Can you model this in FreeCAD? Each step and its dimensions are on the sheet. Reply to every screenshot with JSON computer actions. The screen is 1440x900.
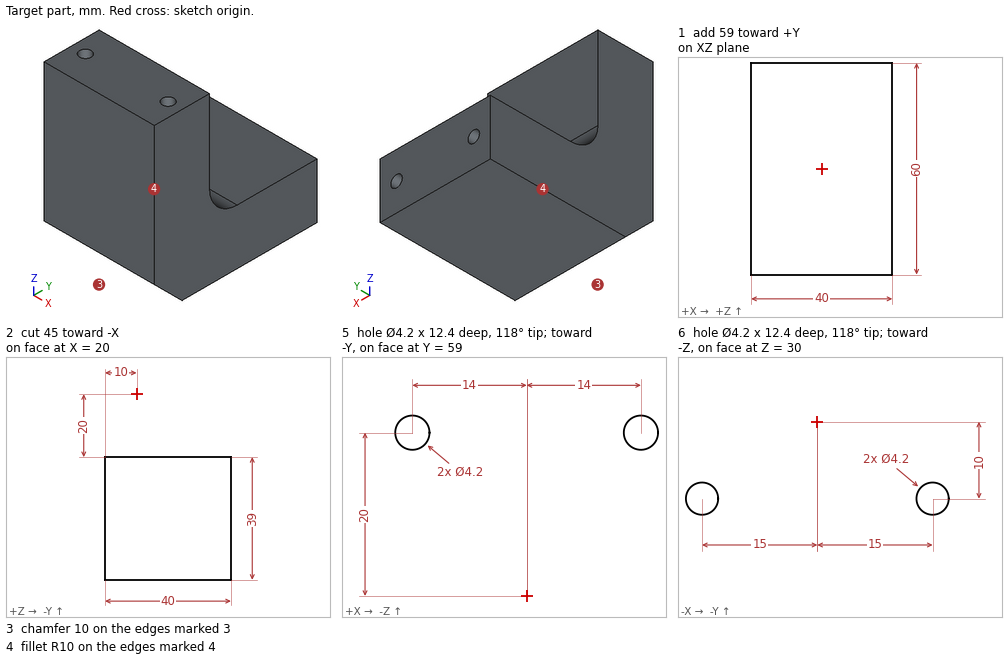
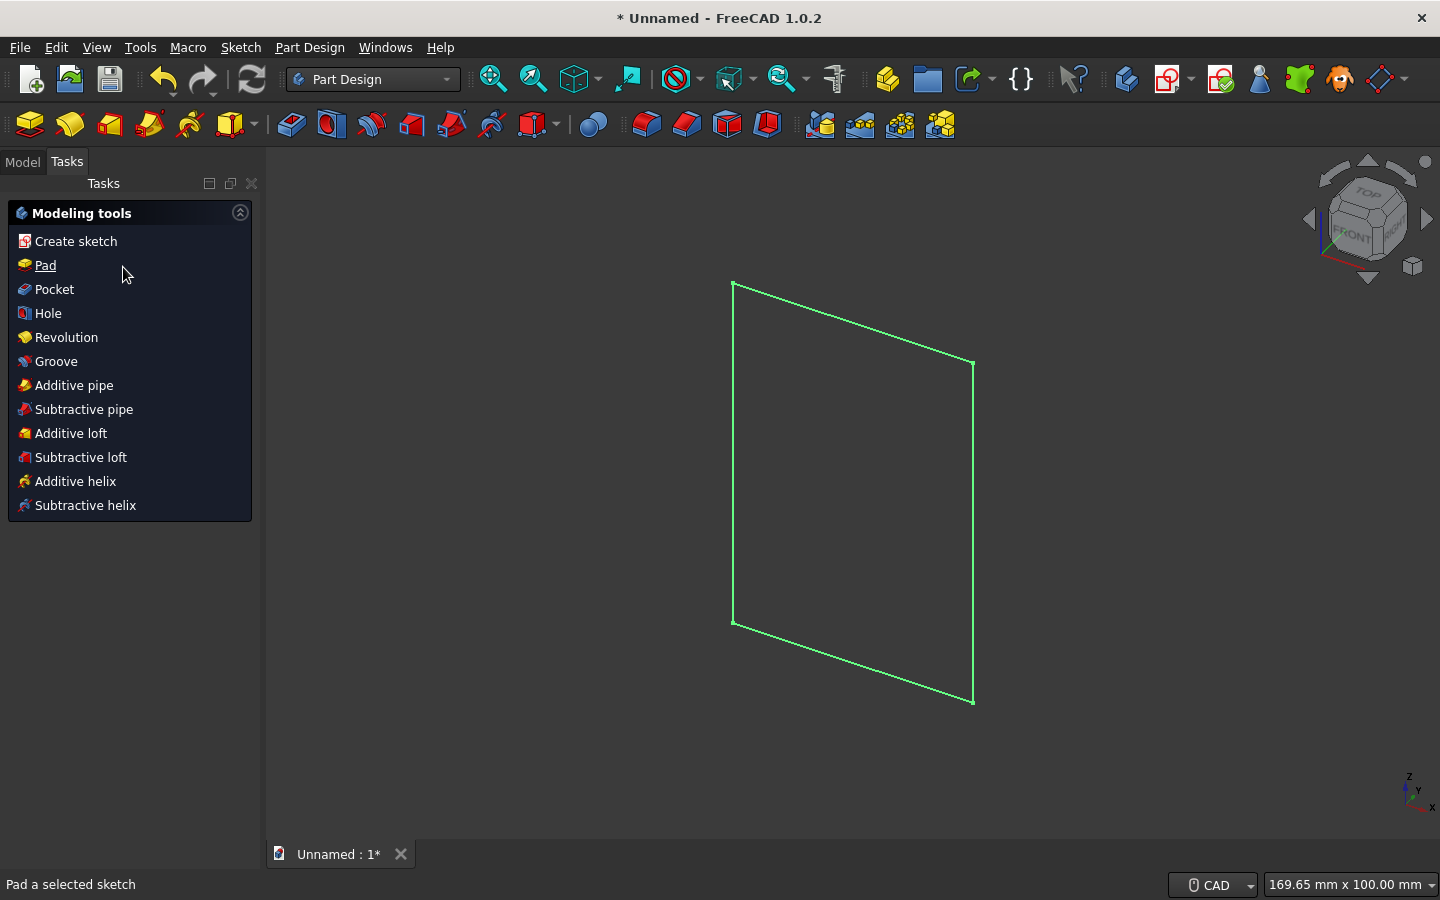
{"action": "left_click", "coordinate": [30, 124]}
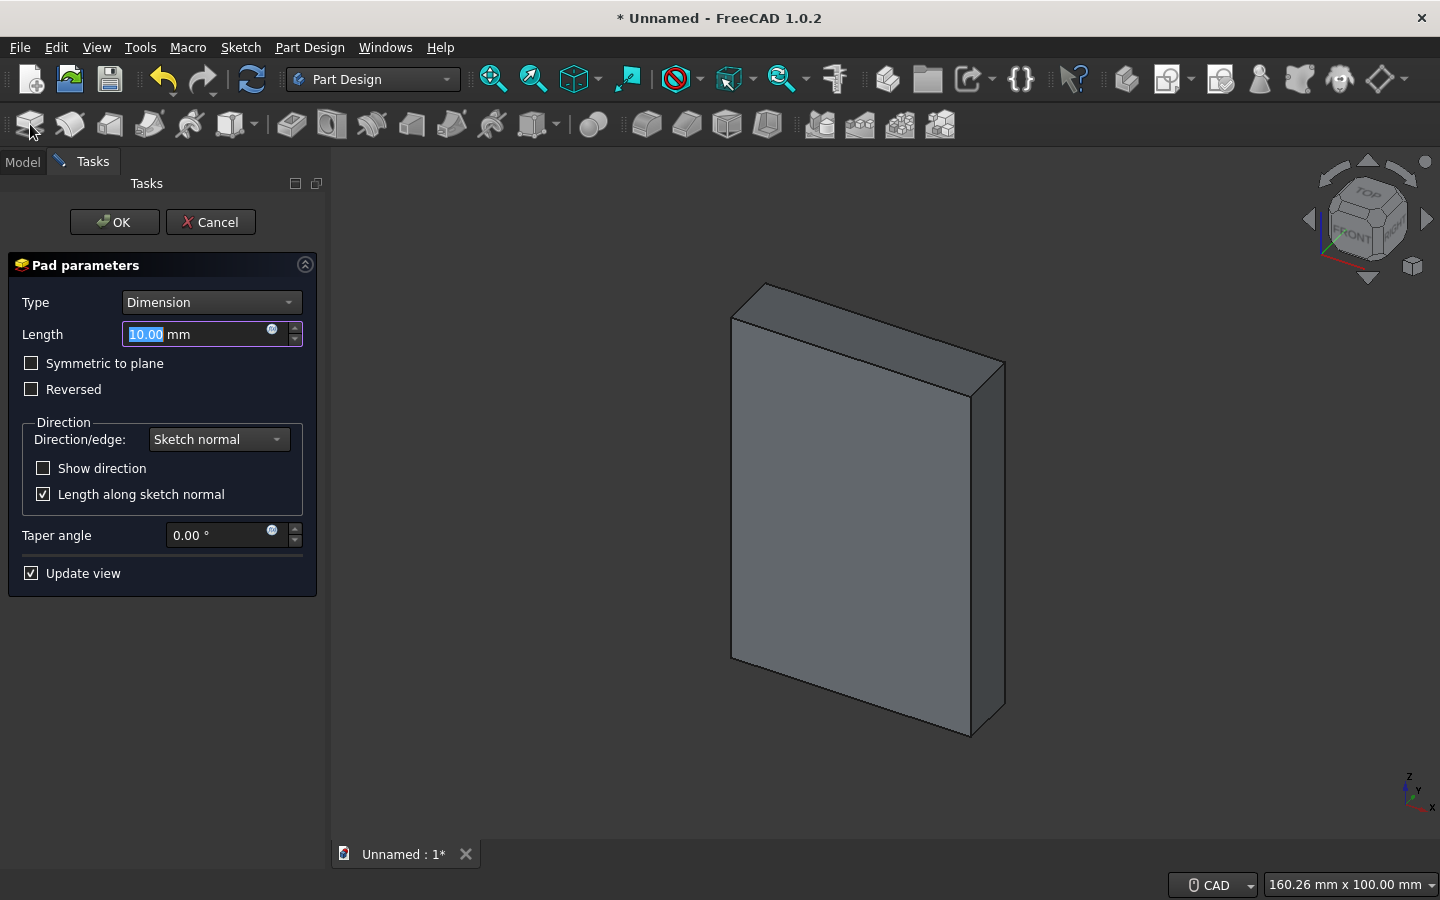
{"action": "type", "text": "59"}
{"action": "key", "text": "Tab"}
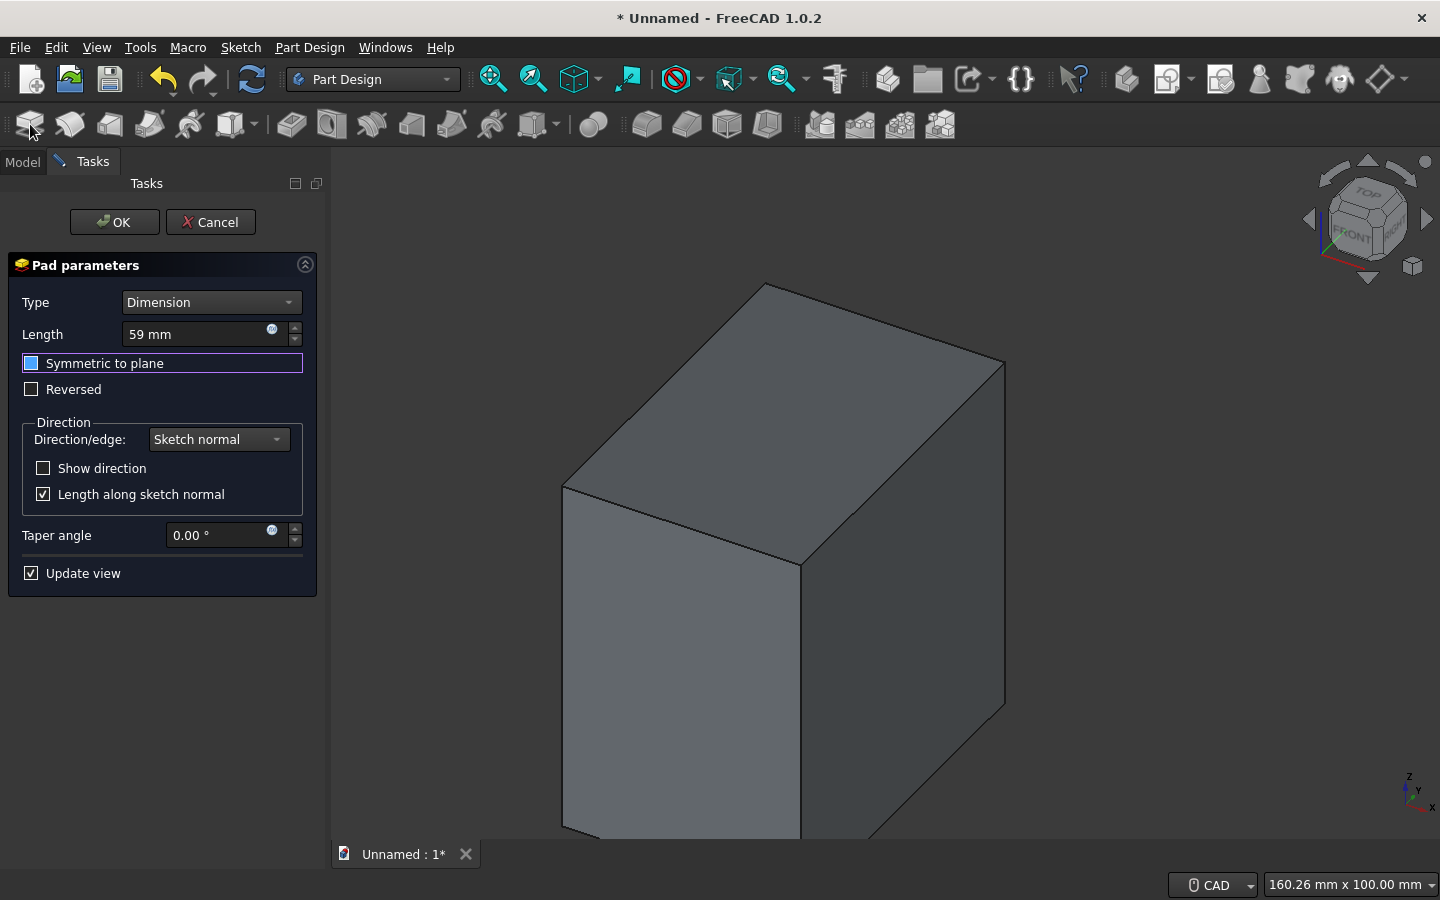
{"action": "left_click", "coordinate": [30, 389]}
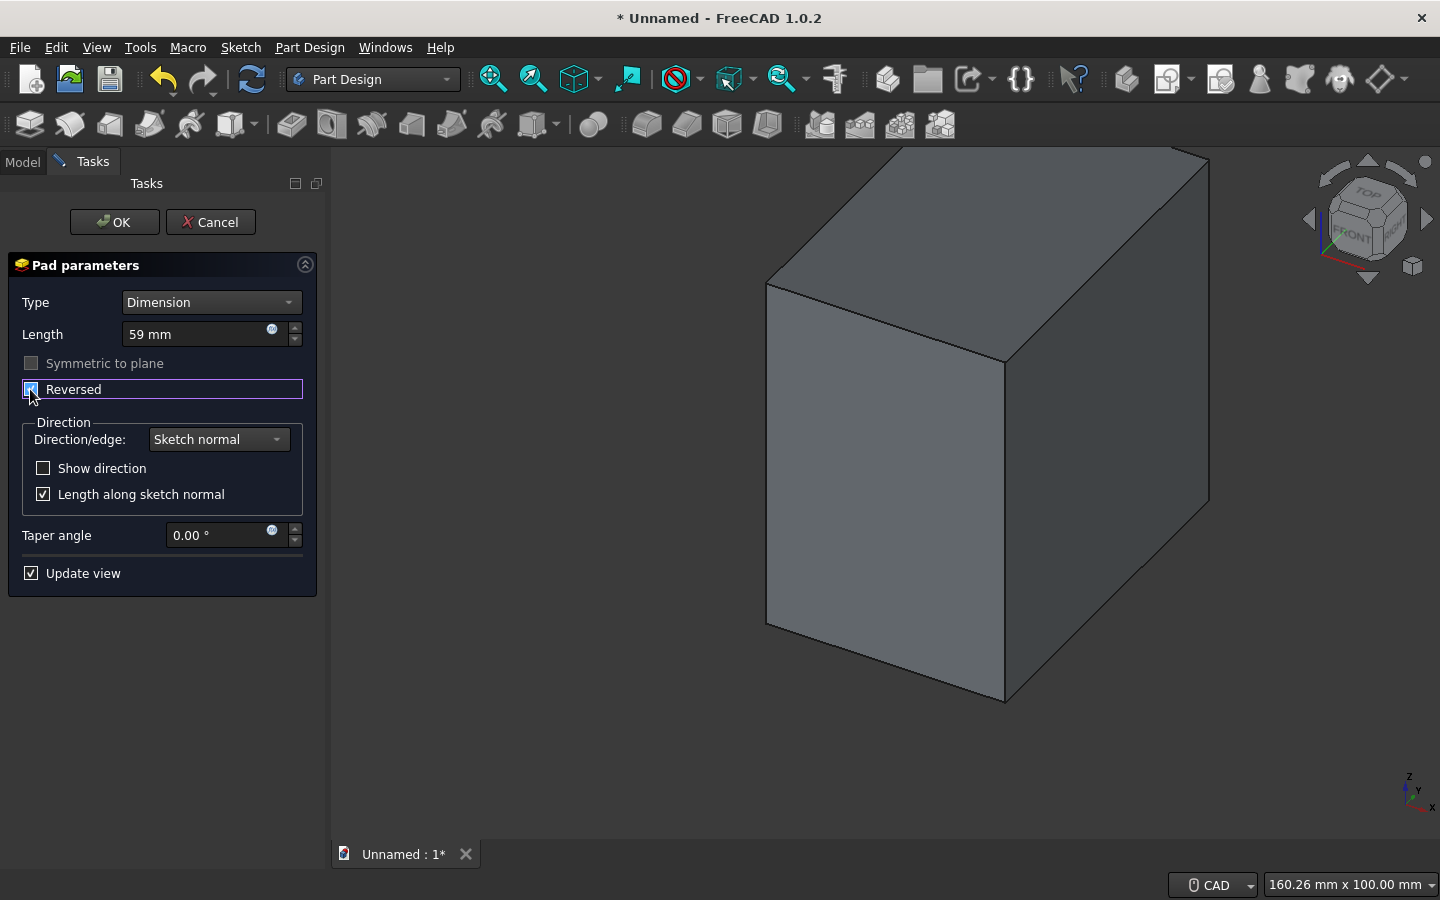
{"action": "left_click", "coordinate": [115, 222]}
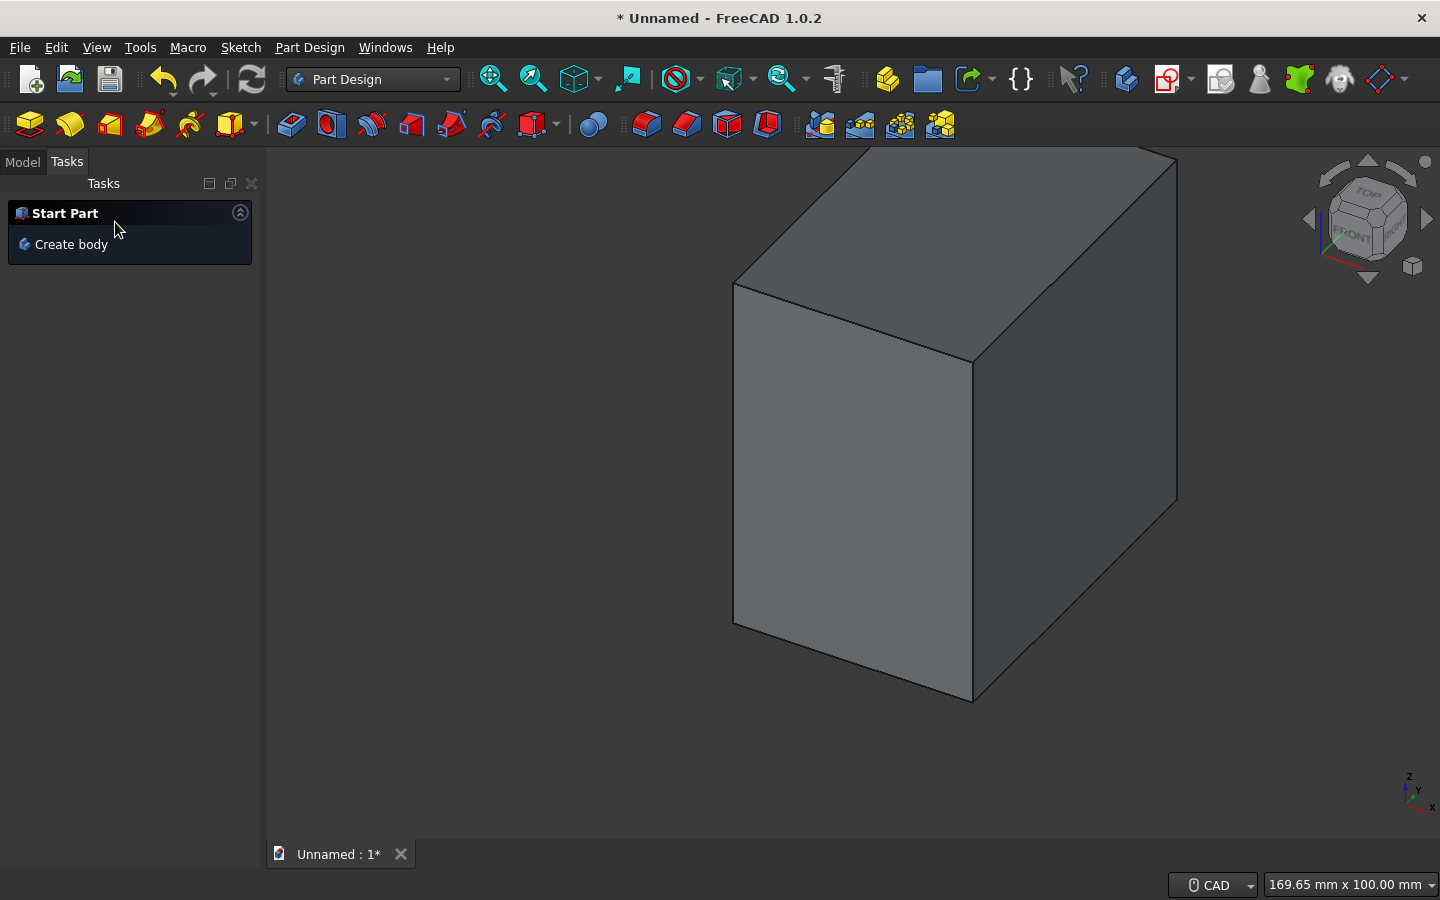
{"action": "left_click", "coordinate": [494, 80]}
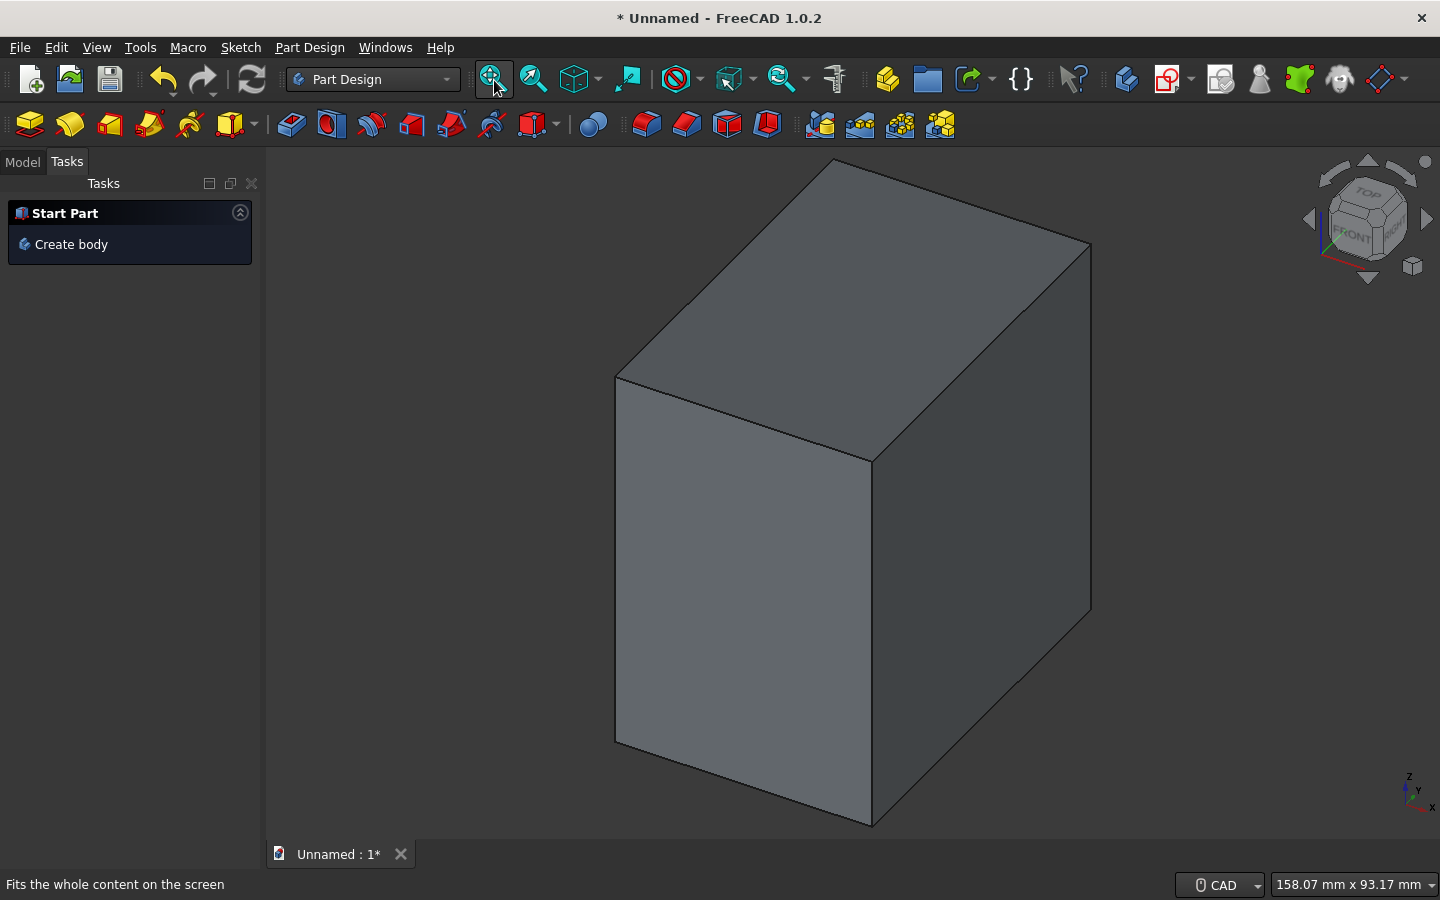
{"action": "left_click", "coordinate": [982, 535]}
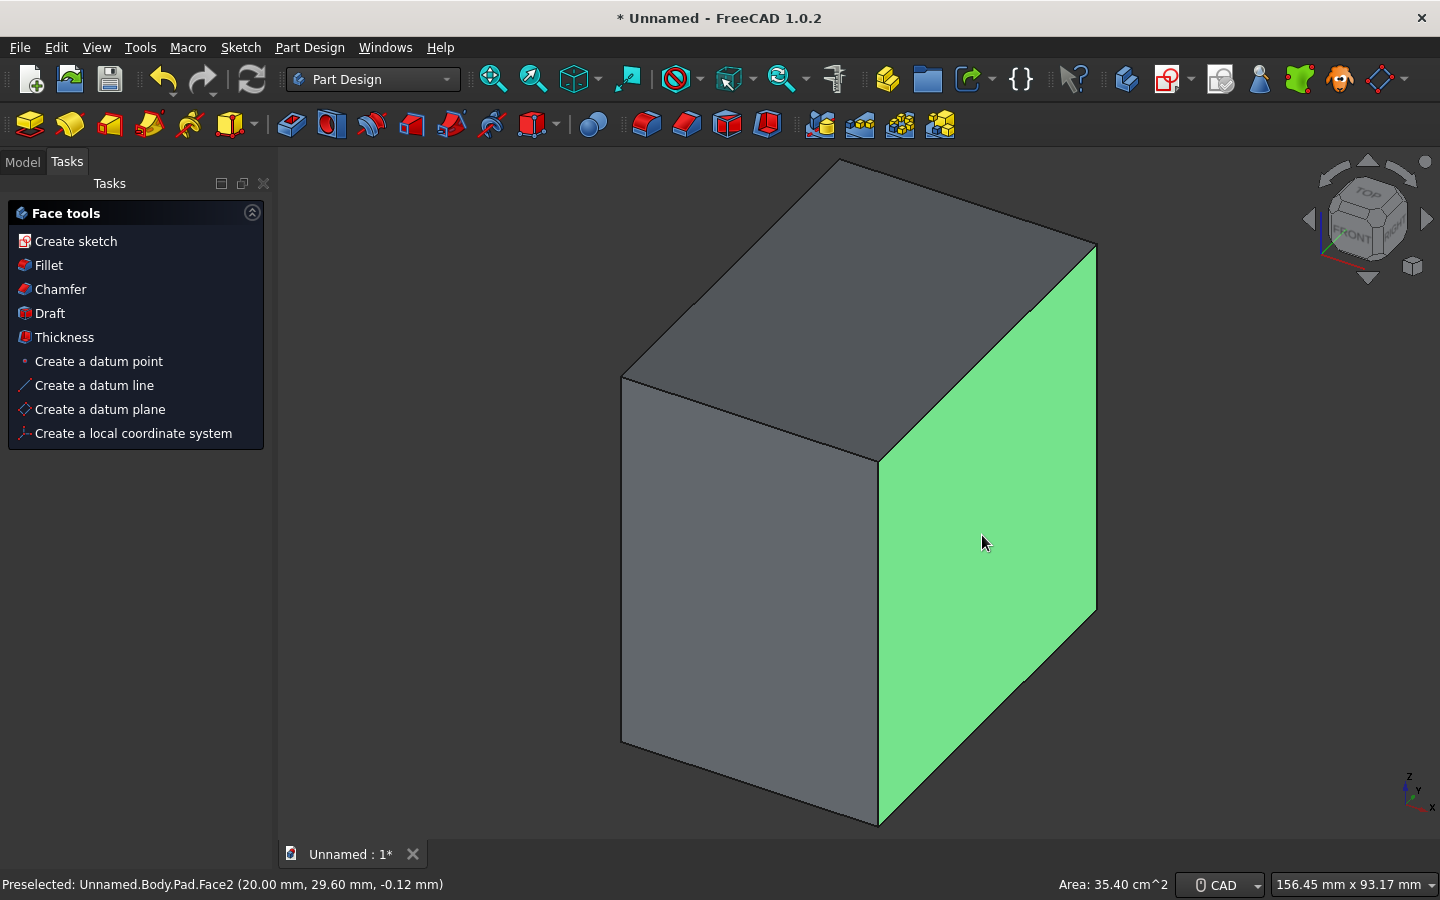
{"action": "left_click", "coordinate": [1168, 80]}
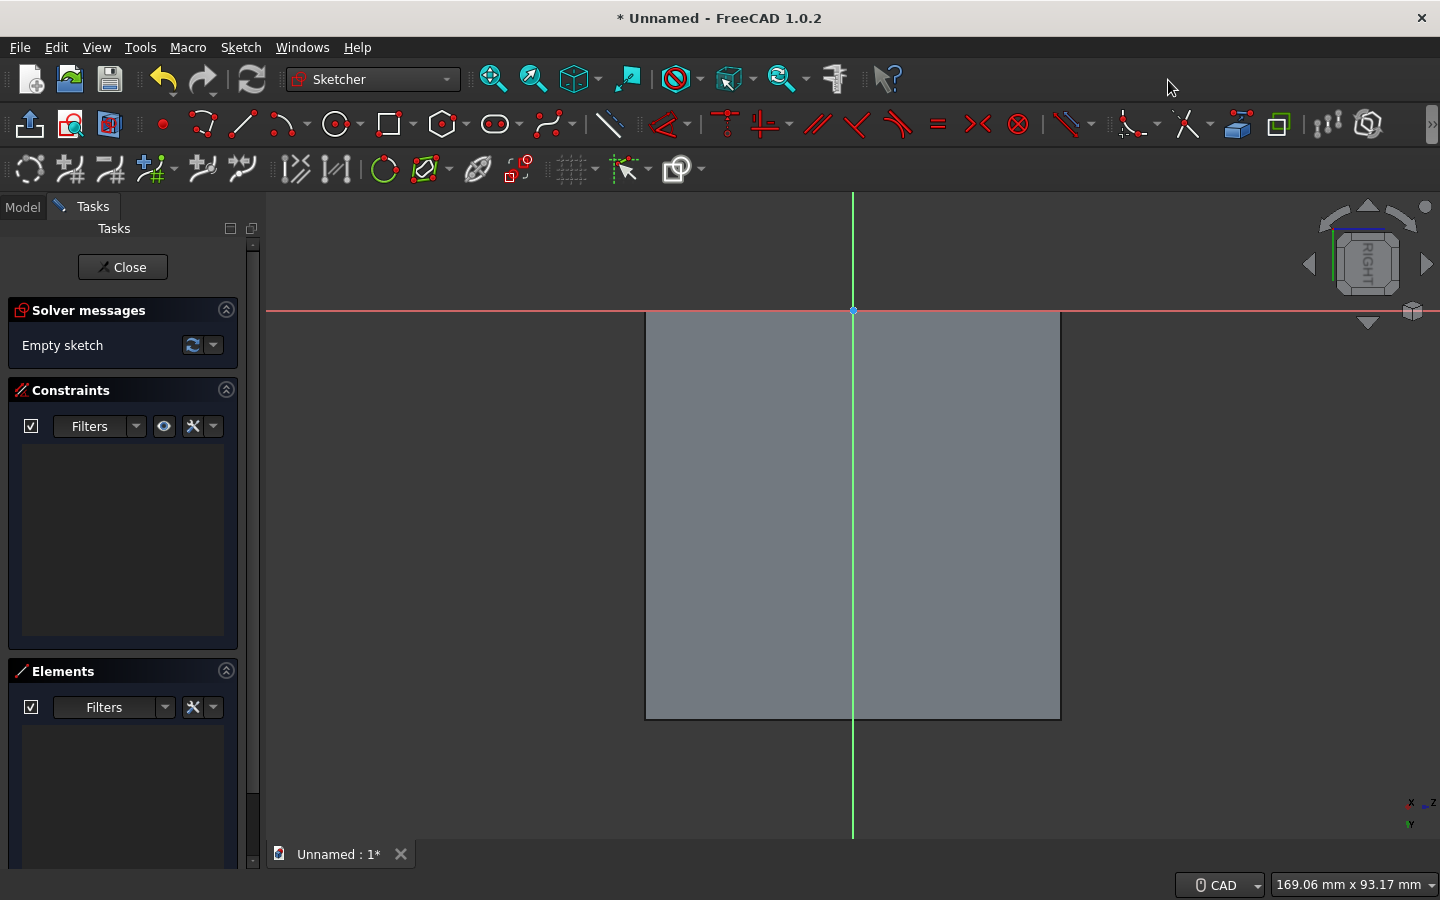
{"action": "left_click", "coordinate": [390, 124]}